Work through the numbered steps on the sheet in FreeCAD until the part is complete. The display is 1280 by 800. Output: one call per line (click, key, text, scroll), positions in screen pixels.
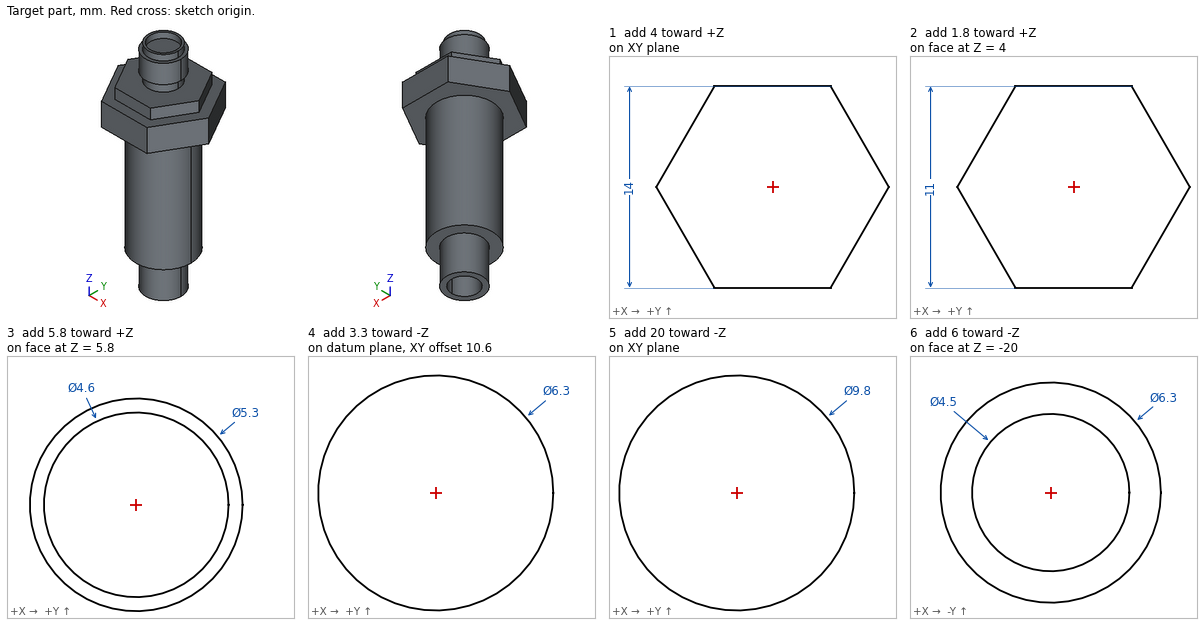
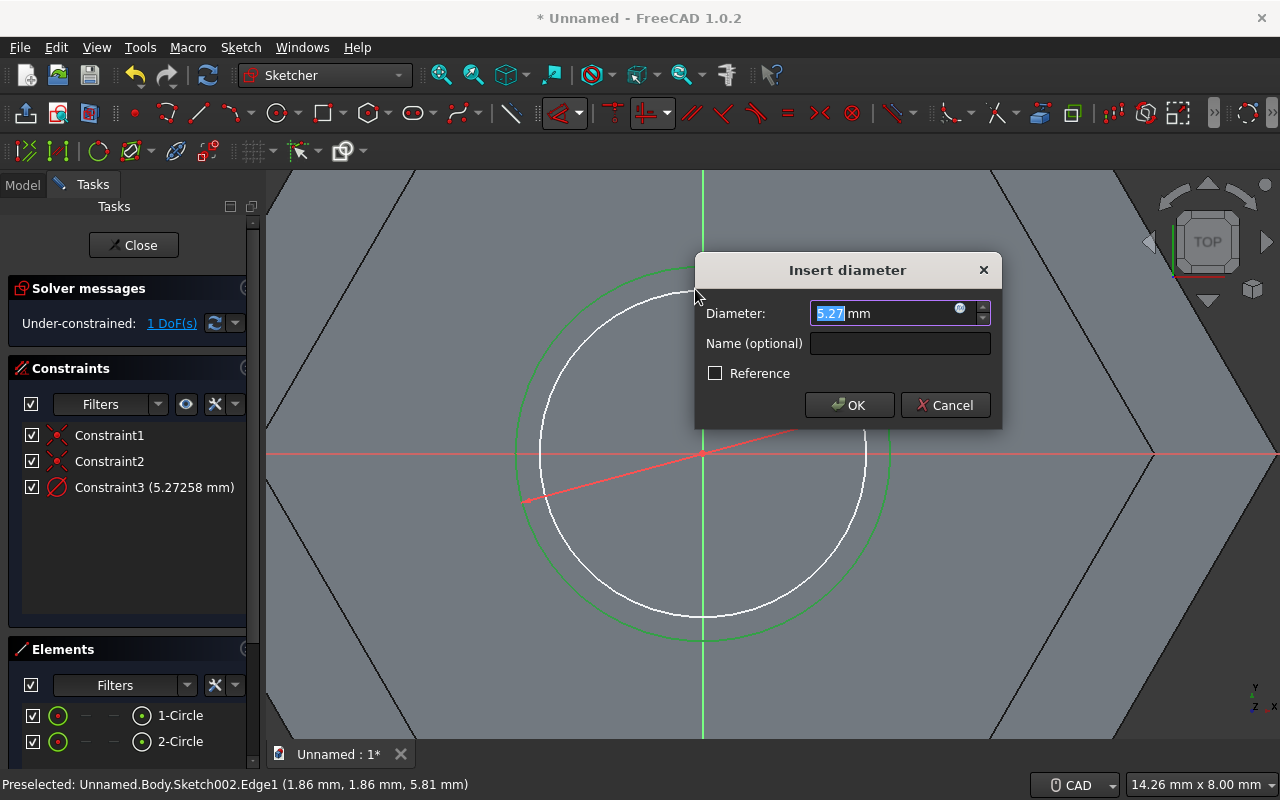
text(5.3)
key(Return)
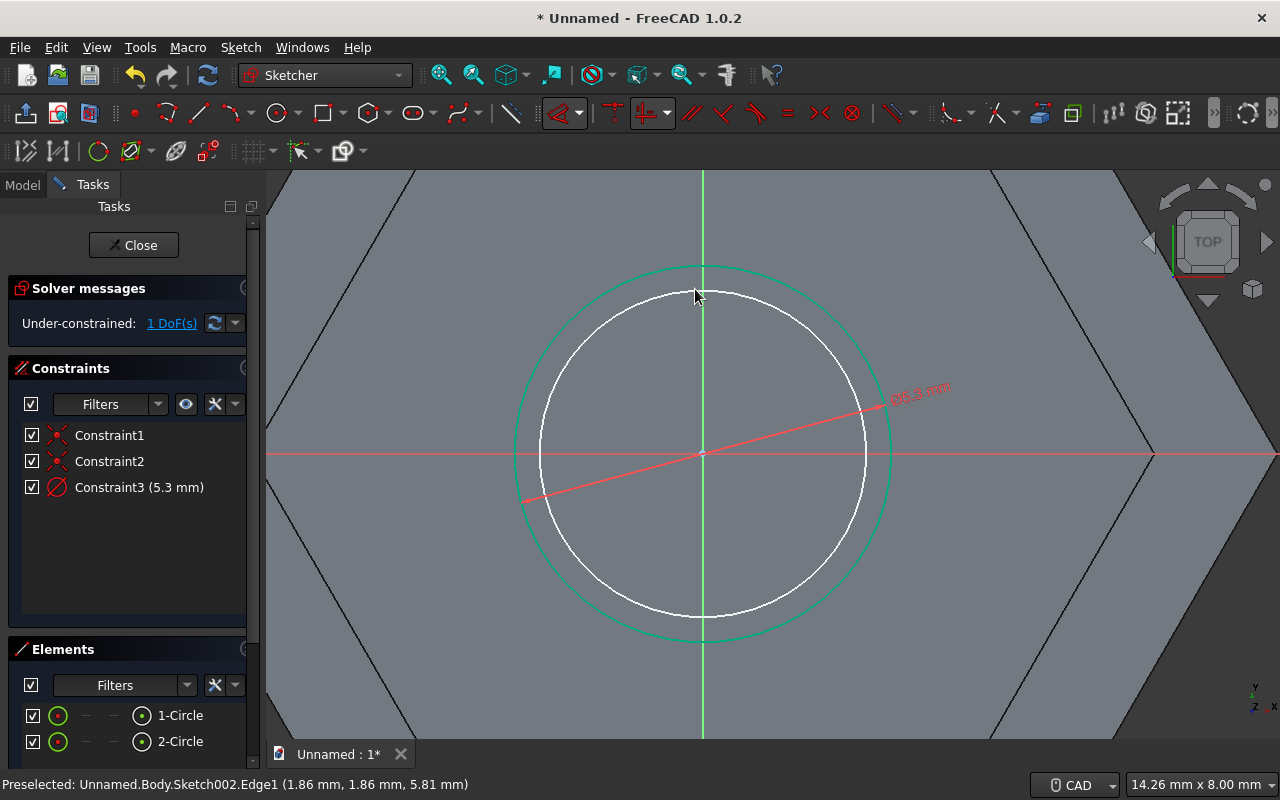
click(818, 338)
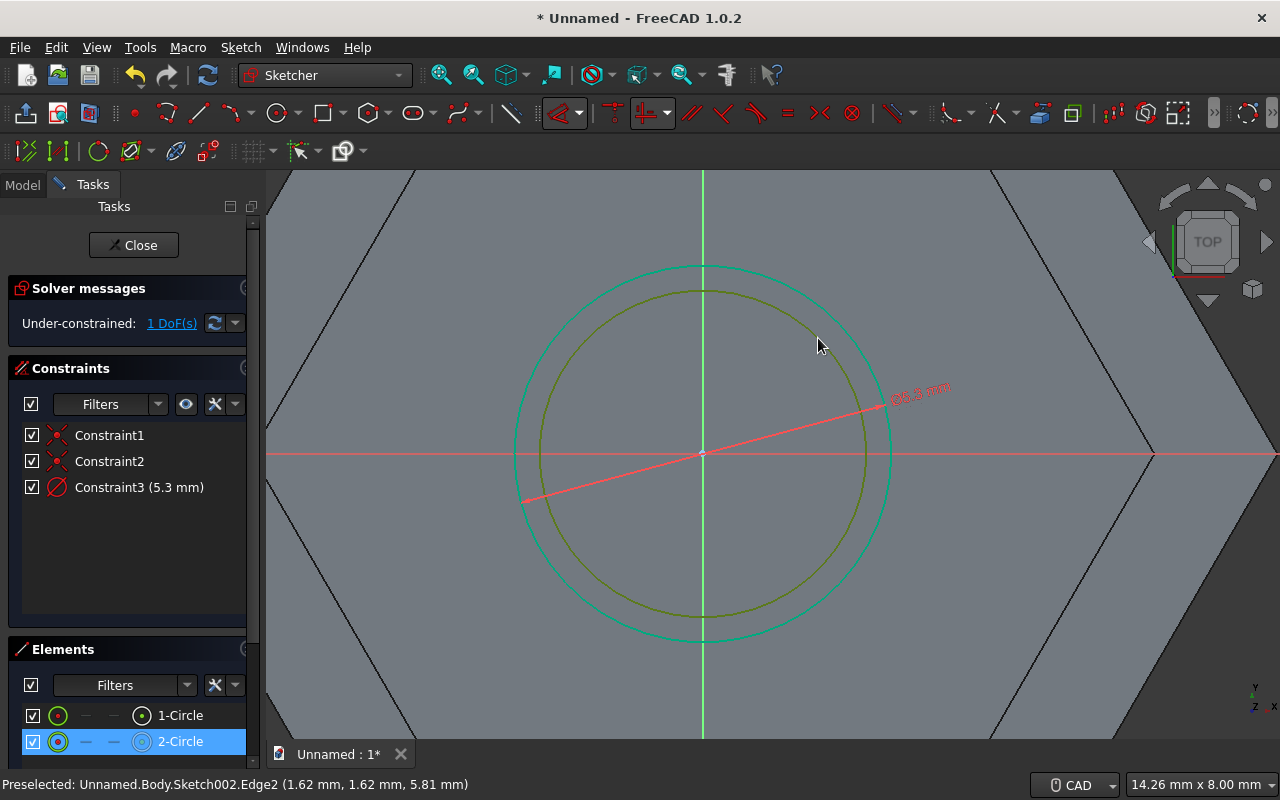
click(582, 114)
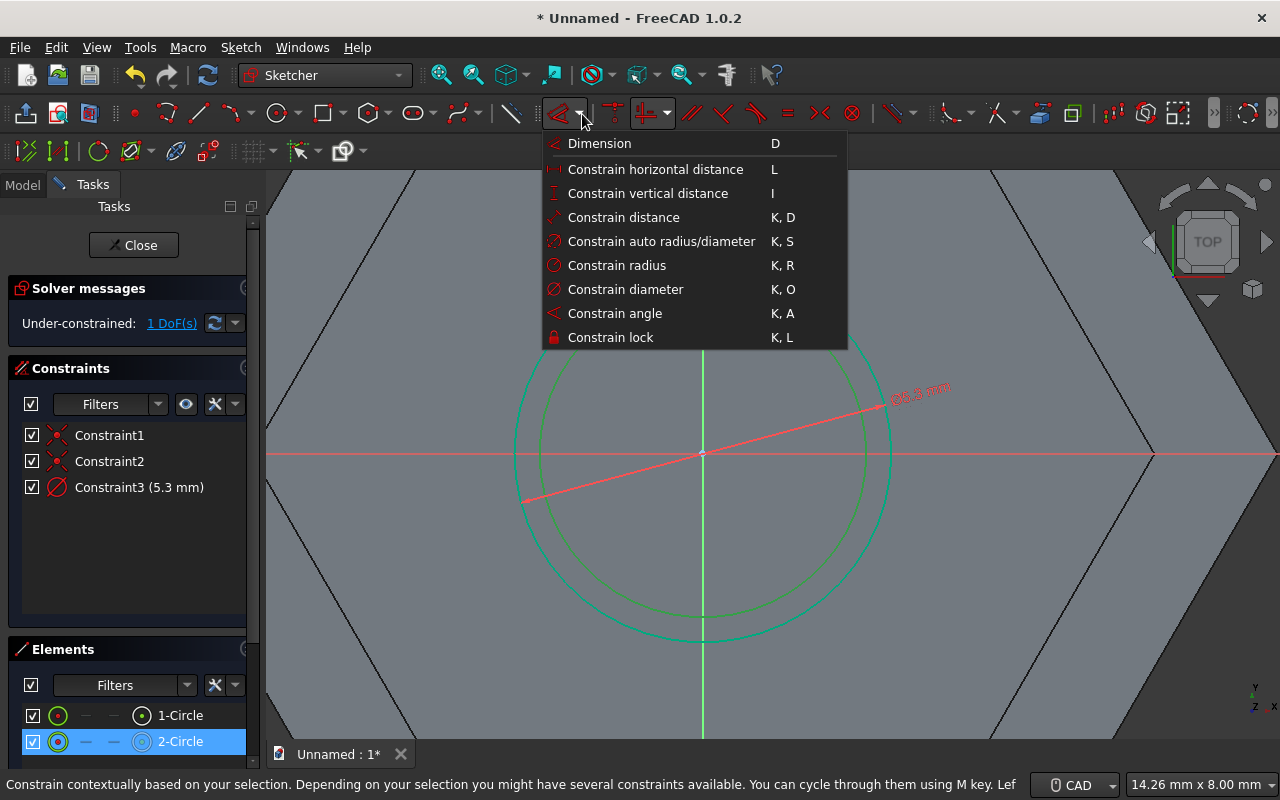
click(695, 289)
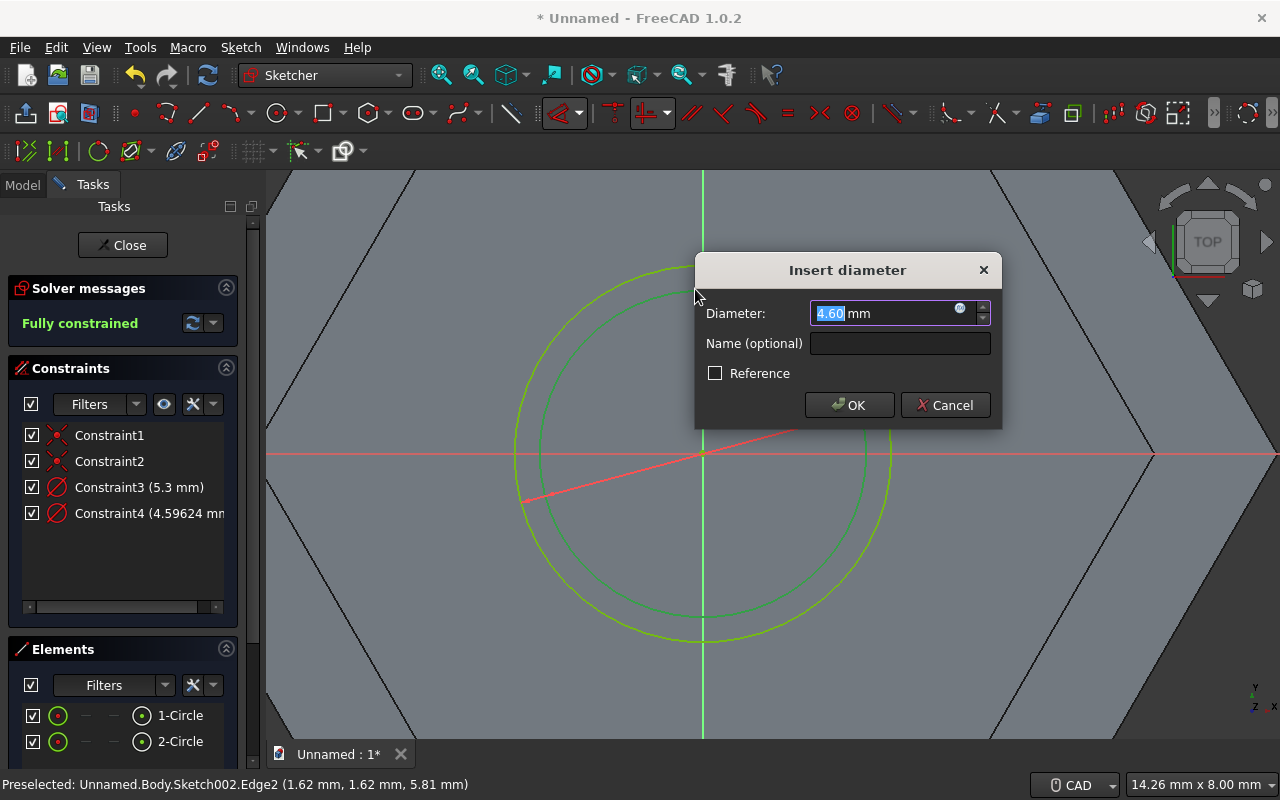
text(4.6)
key(Return)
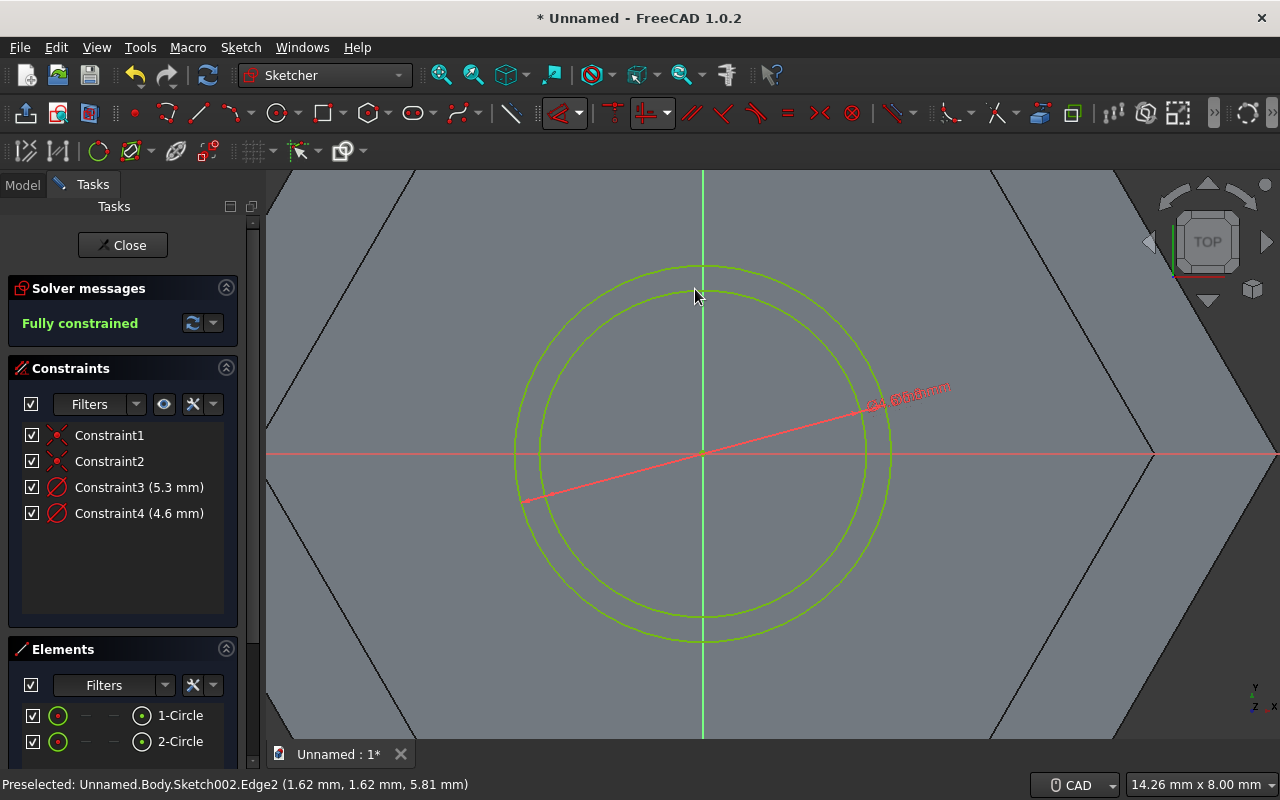
click(123, 245)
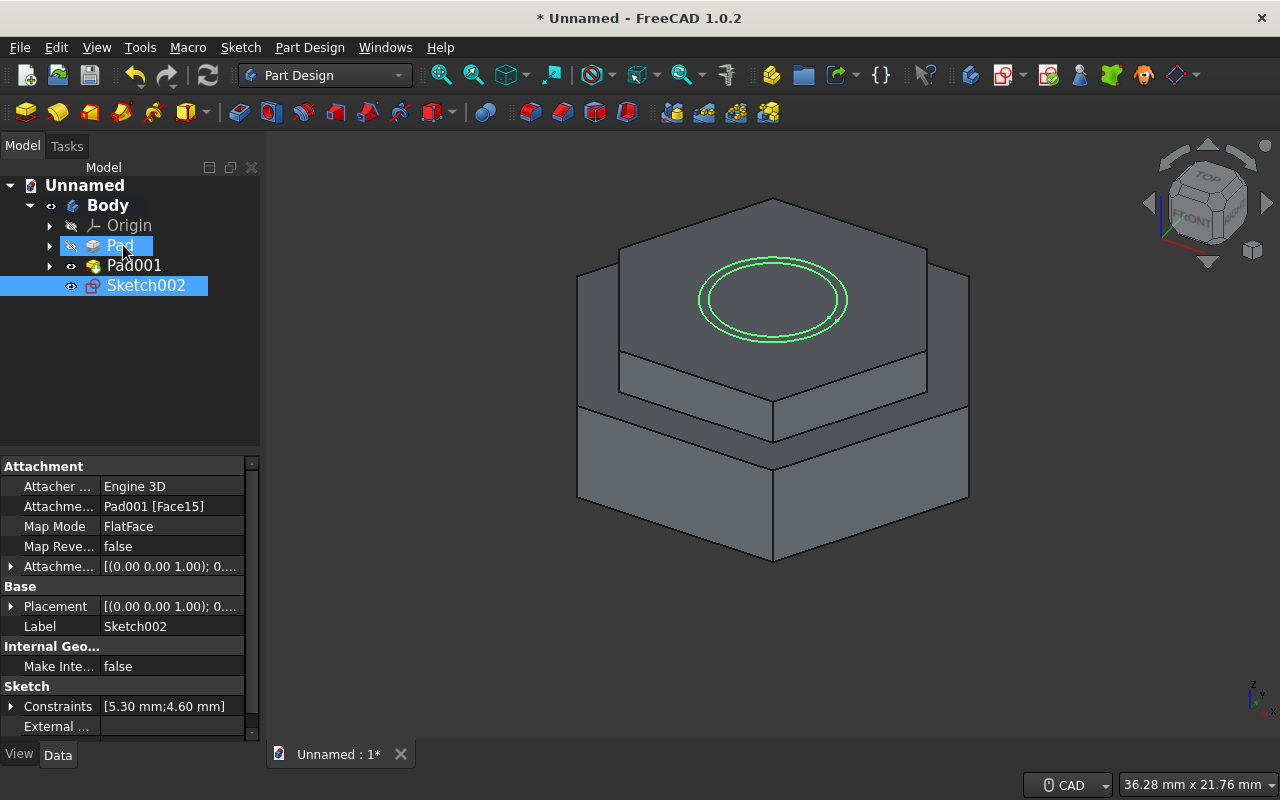
click(26, 112)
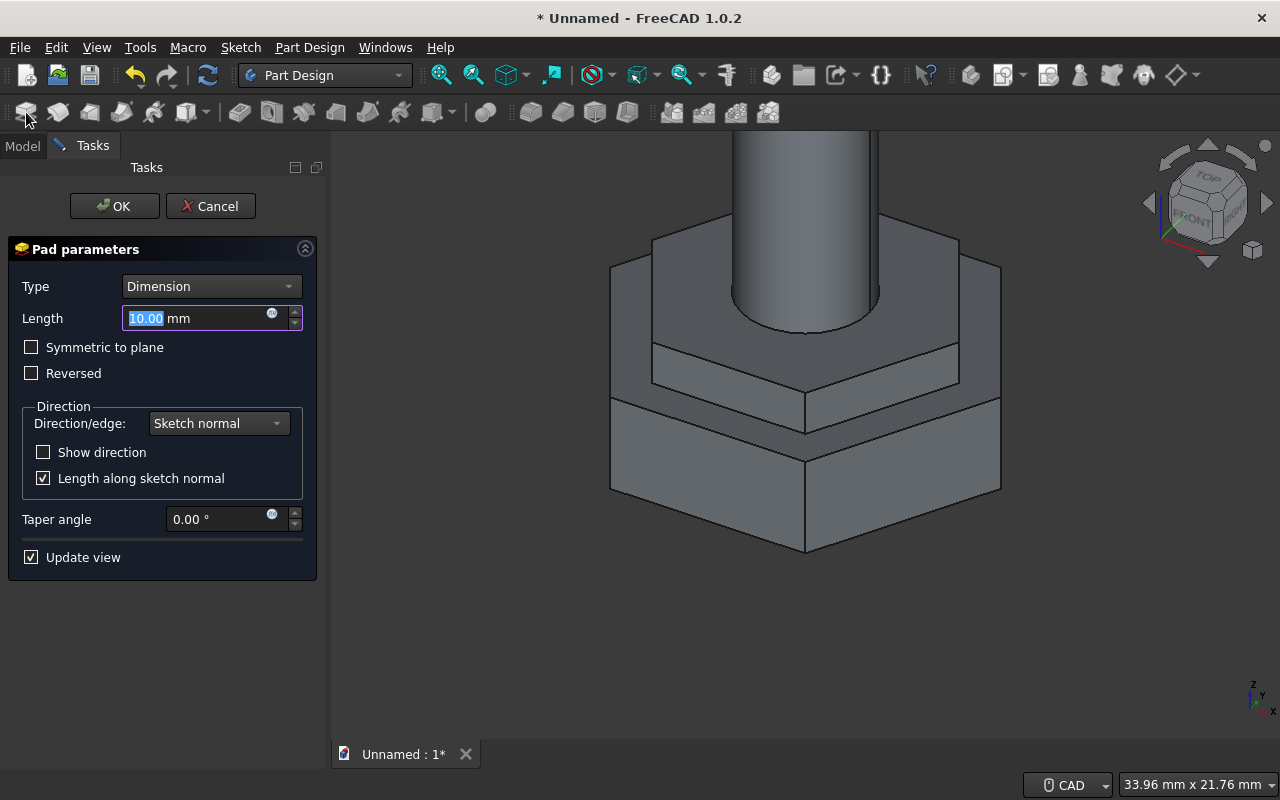
text(5.8)
key(Tab)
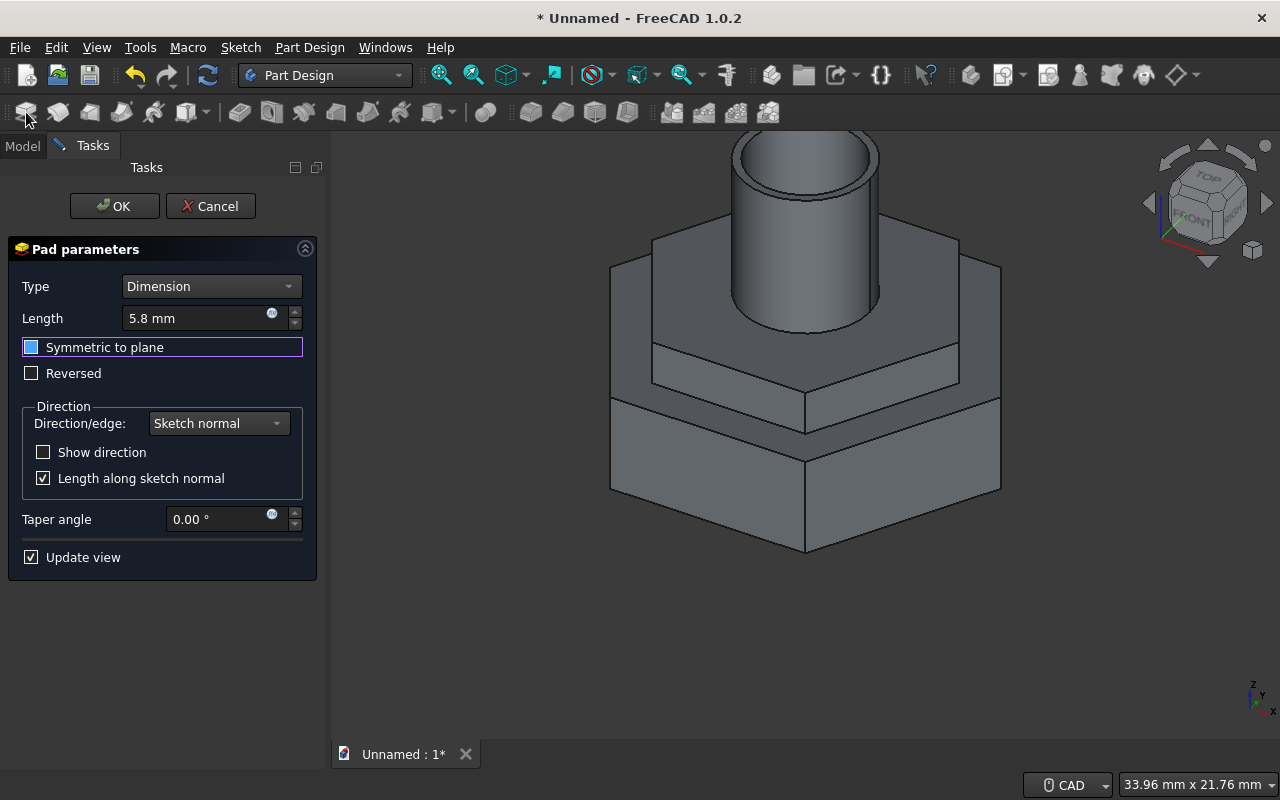
click(115, 206)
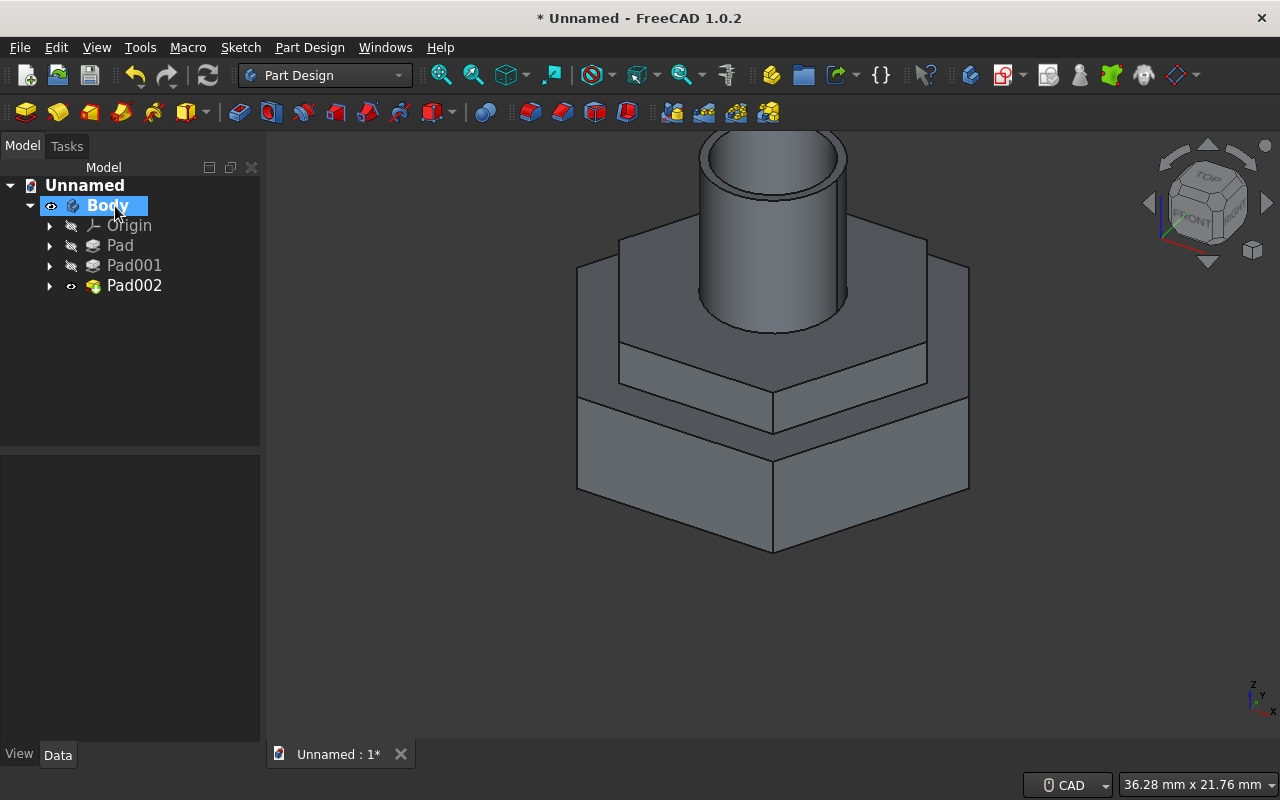
click(442, 76)